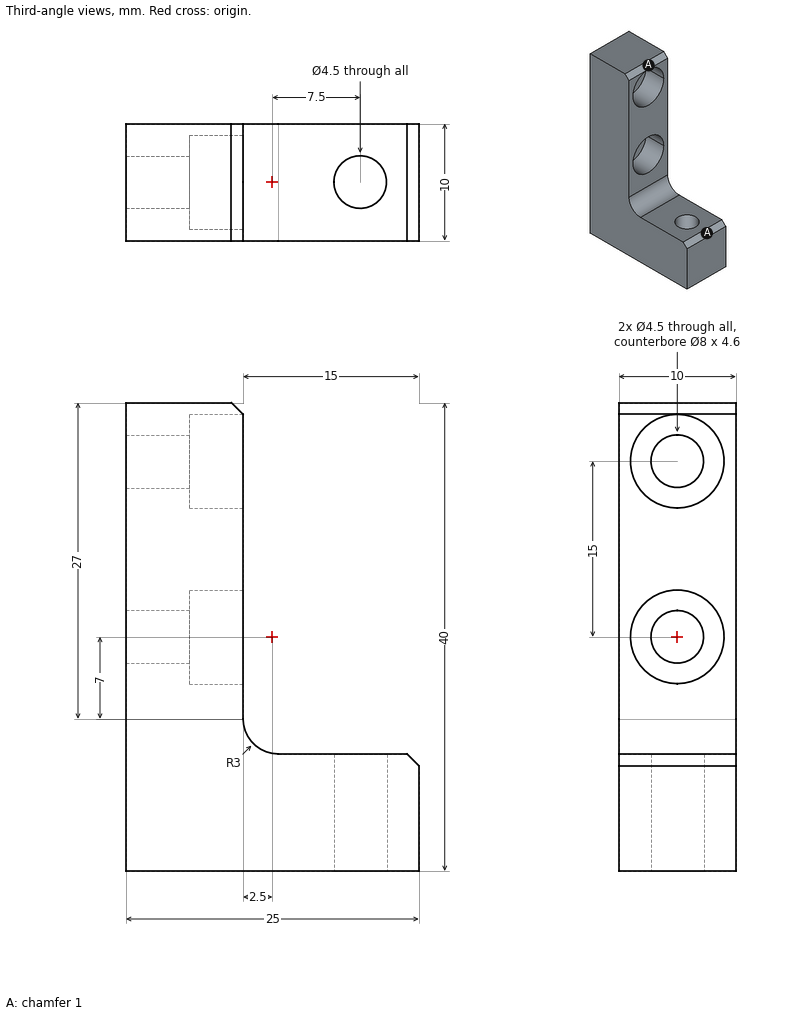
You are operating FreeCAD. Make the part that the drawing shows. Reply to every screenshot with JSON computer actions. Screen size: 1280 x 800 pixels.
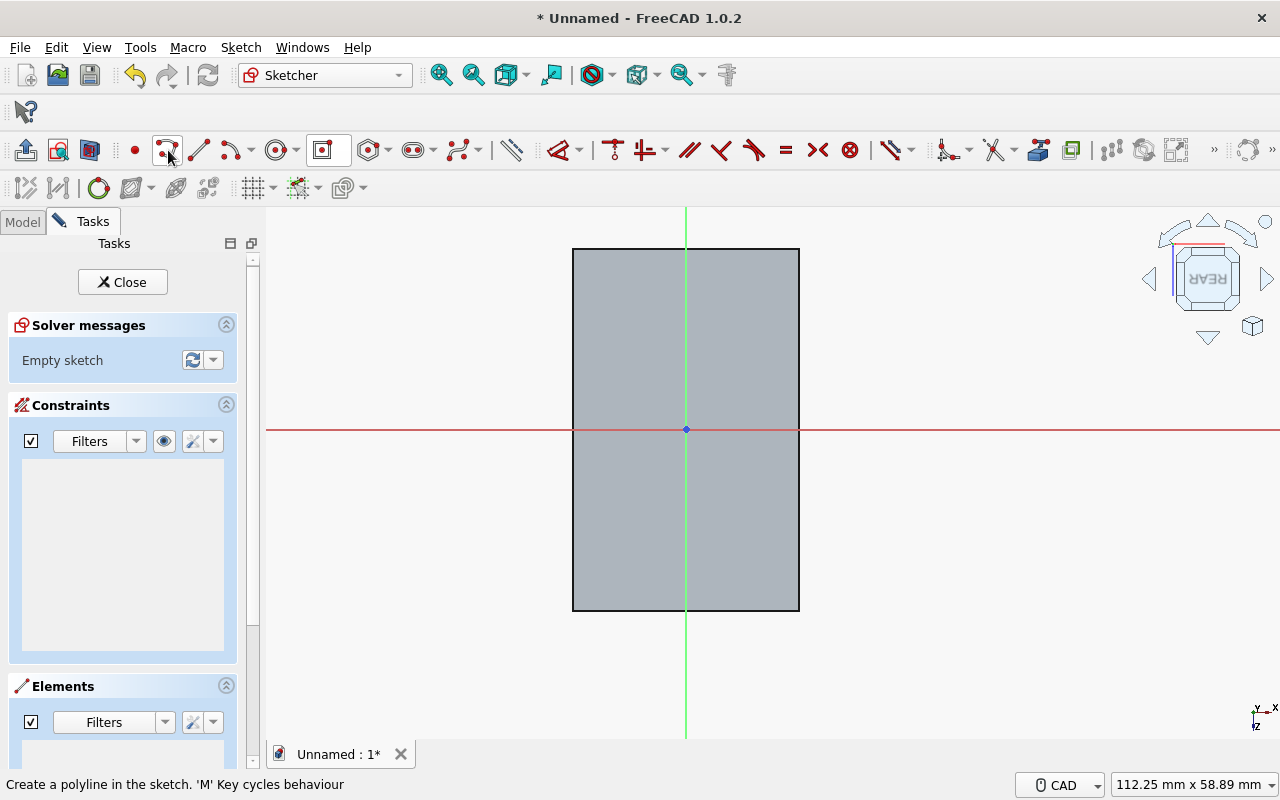
{"action": "left_click", "coordinate": [664, 367]}
{"action": "left_click", "coordinate": [664, 611]}
{"action": "left_click", "coordinate": [799, 611]}
{"action": "left_click", "coordinate": [799, 340]}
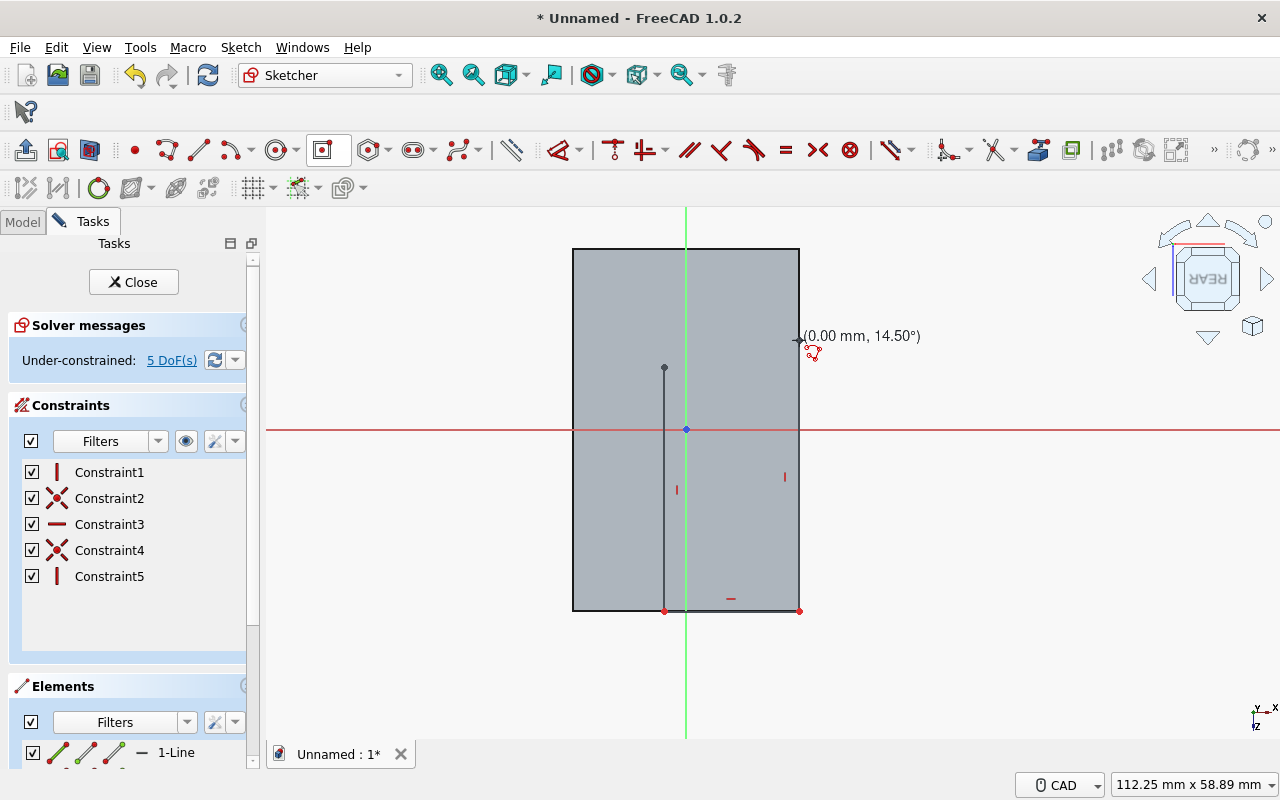
{"action": "scroll", "coordinate": [691, 340], "scroll_direction": "up", "scroll_amount": 7}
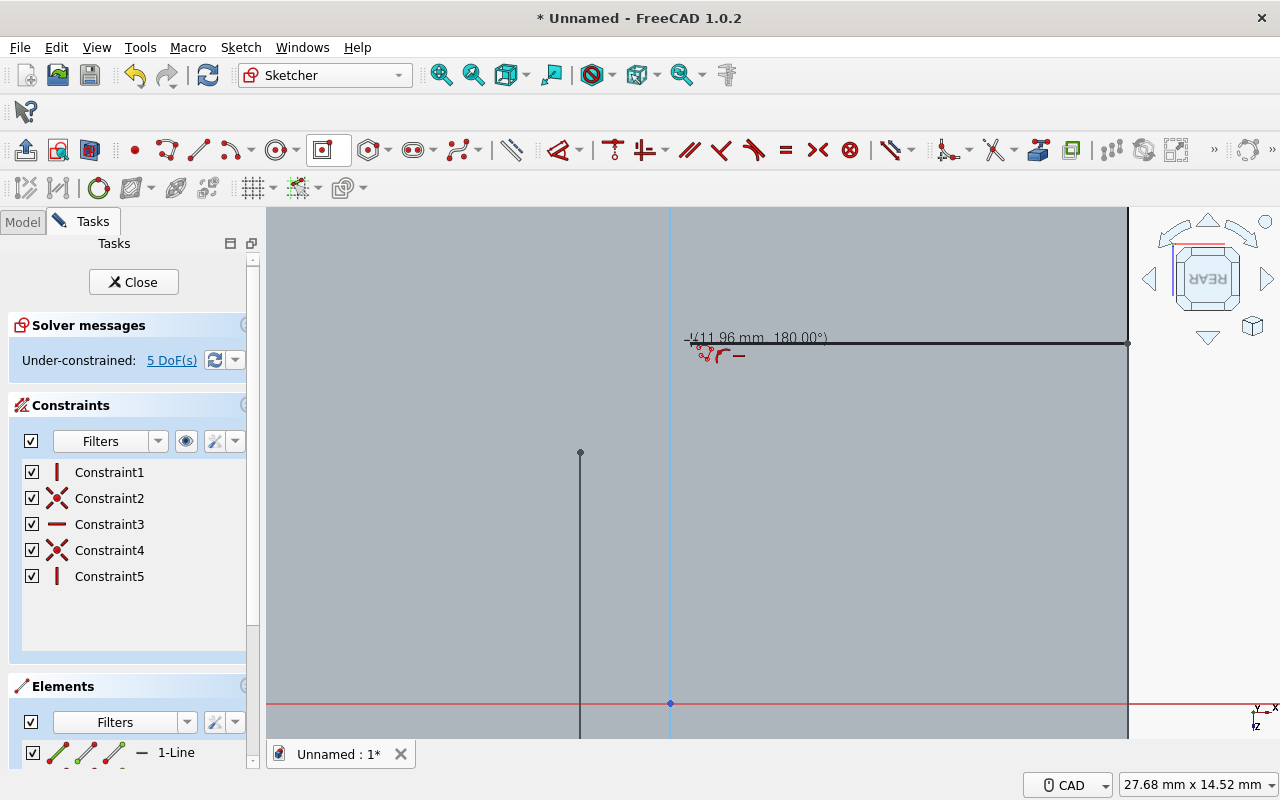
{"action": "left_click", "coordinate": [688, 339]}
{"action": "right_click", "coordinate": [688, 339]}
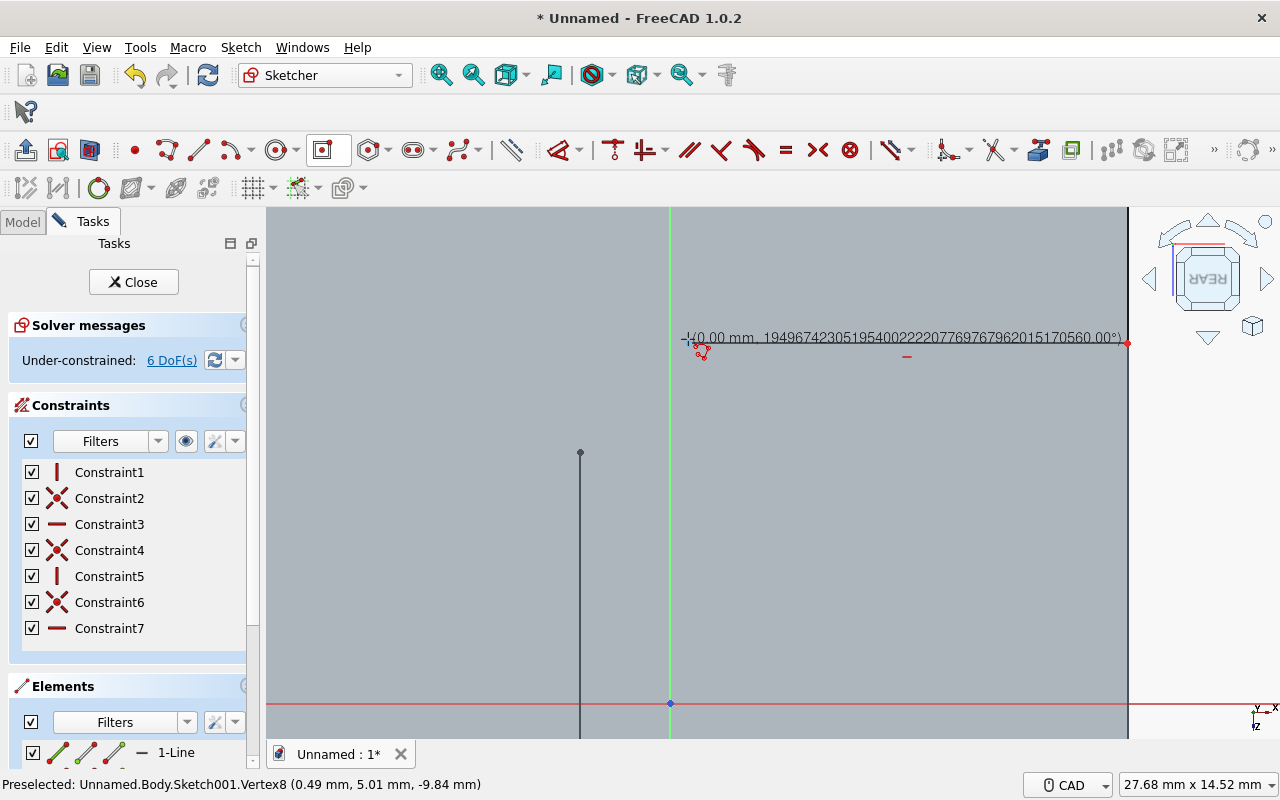
{"action": "left_click", "coordinate": [254, 150]}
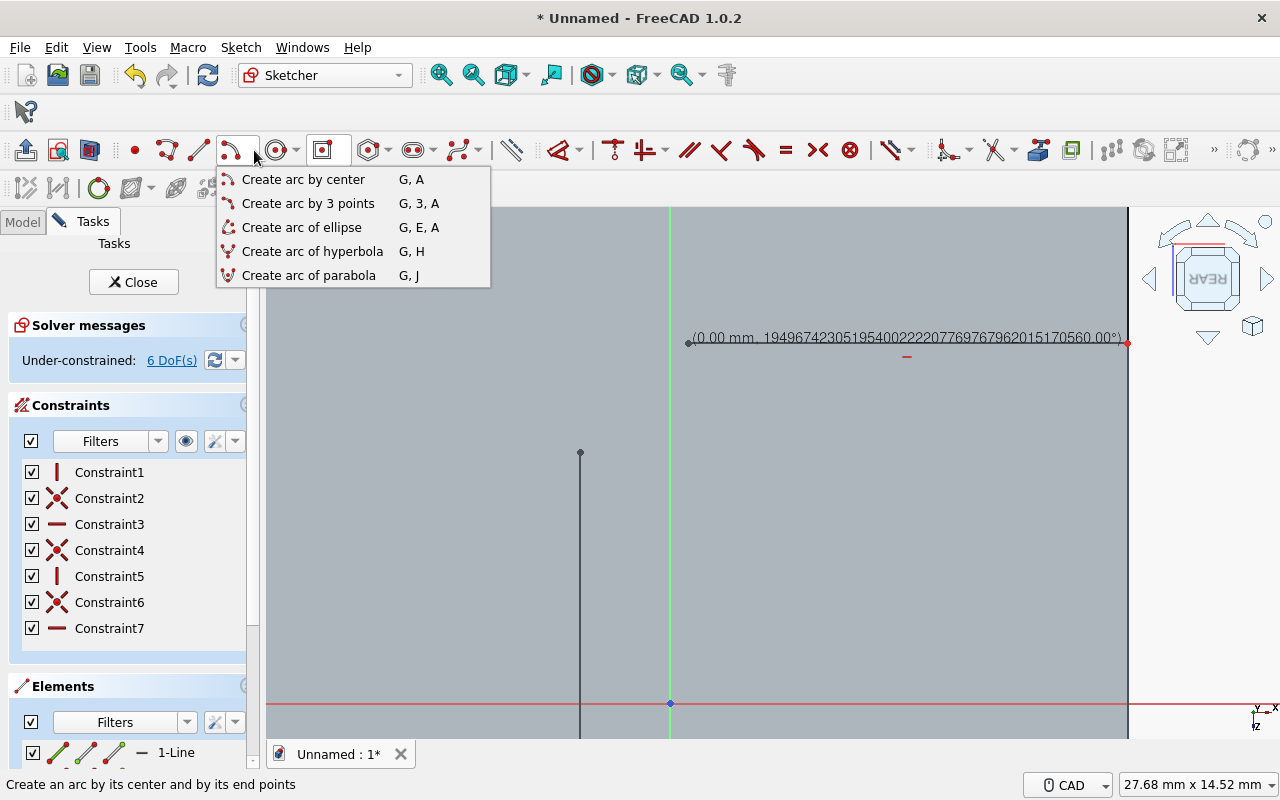
{"action": "left_click", "coordinate": [354, 203]}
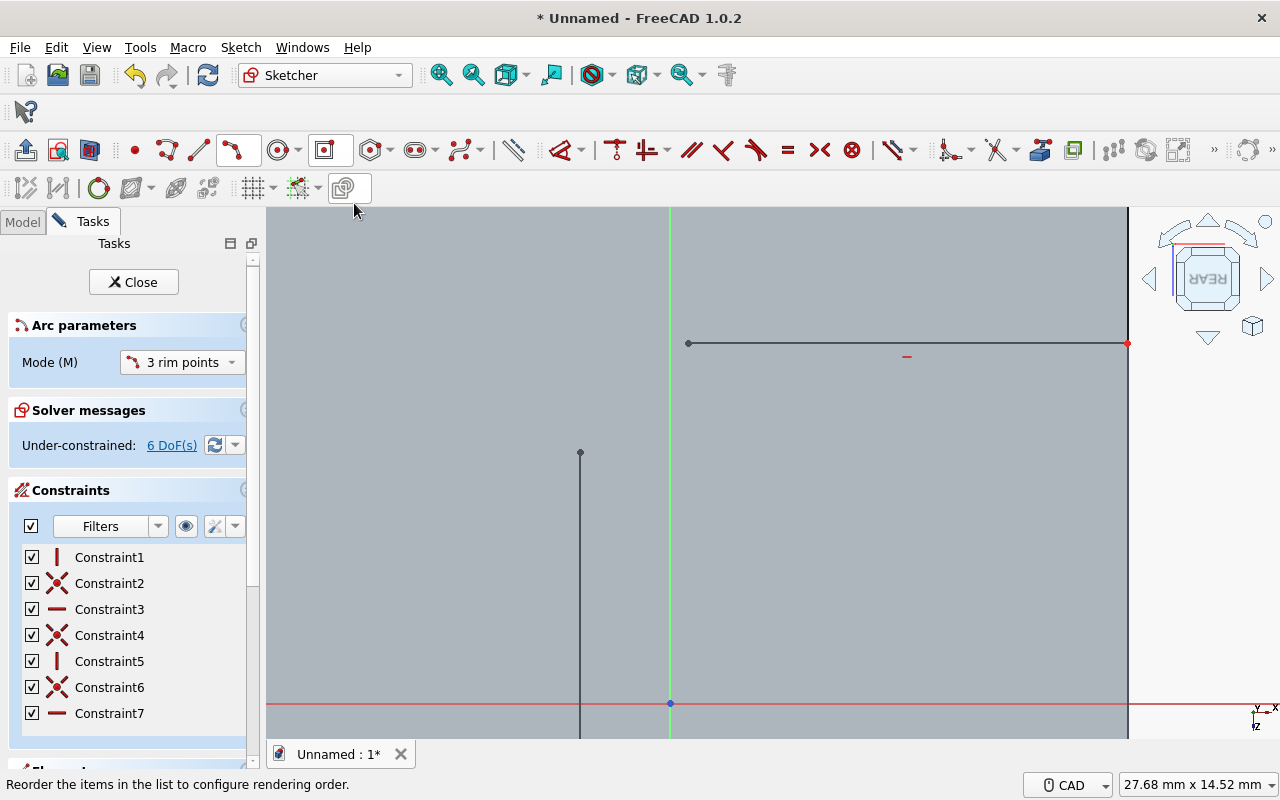
{"action": "left_click", "coordinate": [688, 343]}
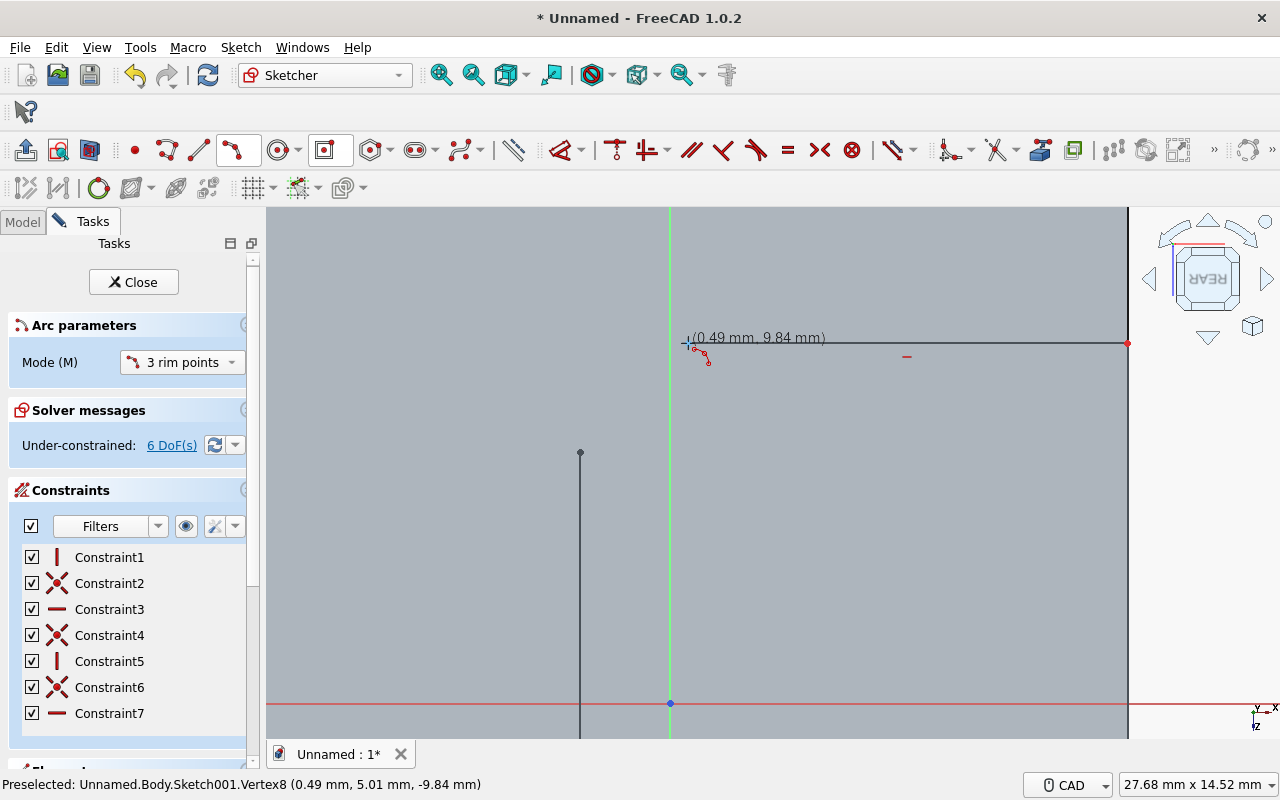
{"action": "scroll", "coordinate": [640, 295], "scroll_direction": "down", "scroll_amount": 6}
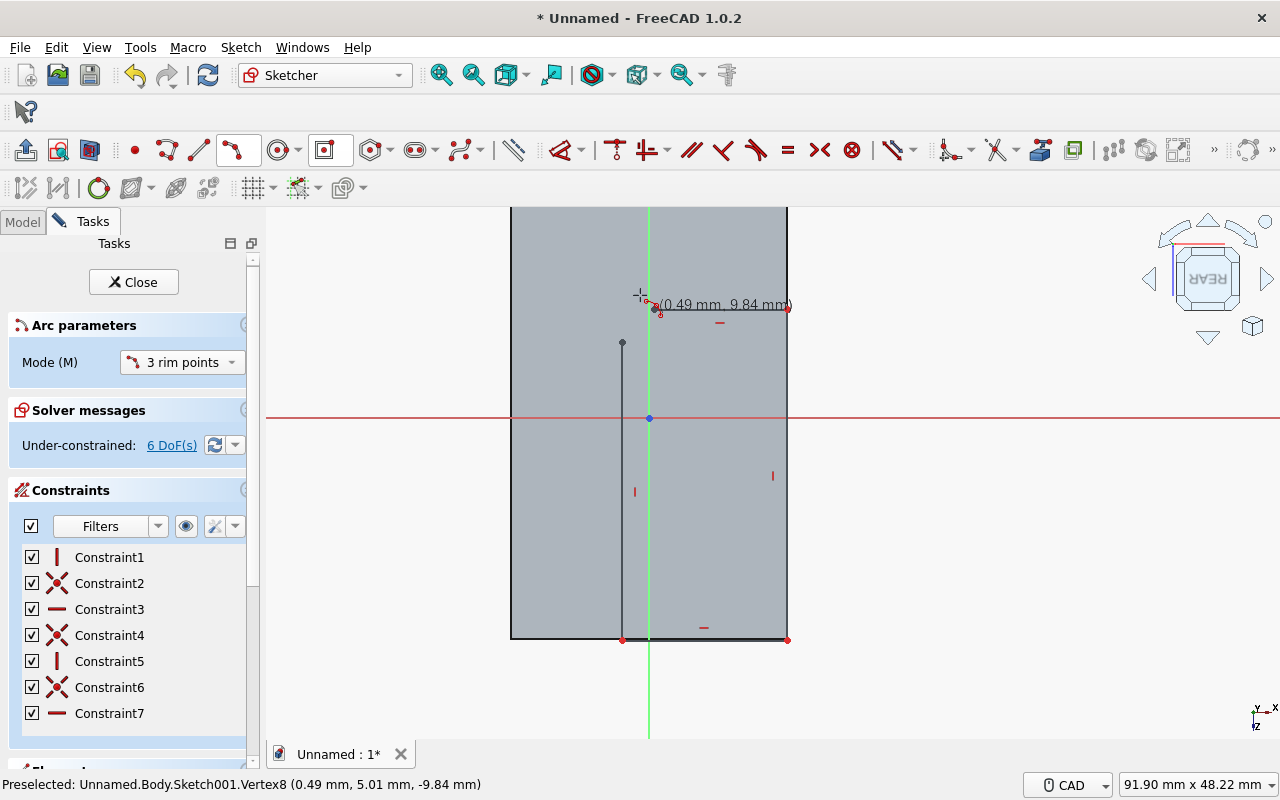
{"action": "left_click", "coordinate": [622, 343]}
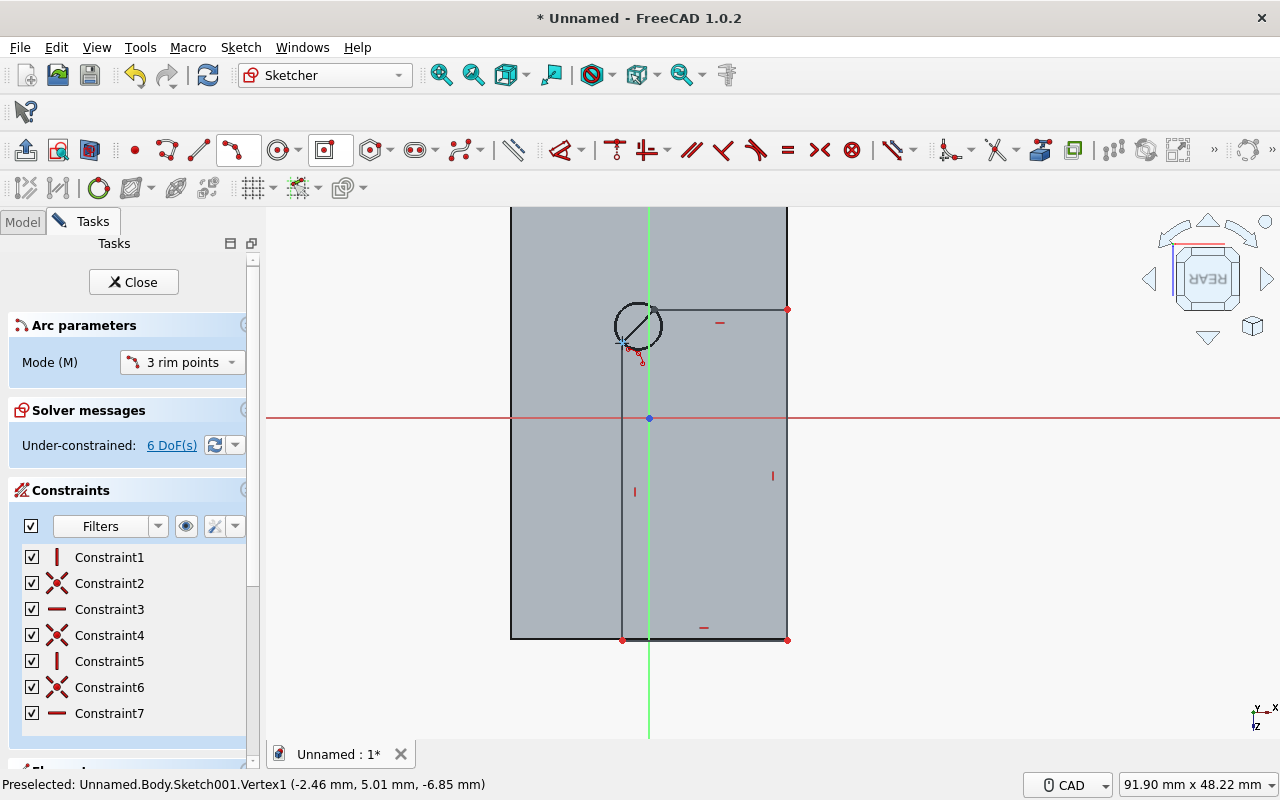
{"action": "scroll", "coordinate": [631, 318], "scroll_direction": "up", "scroll_amount": 3}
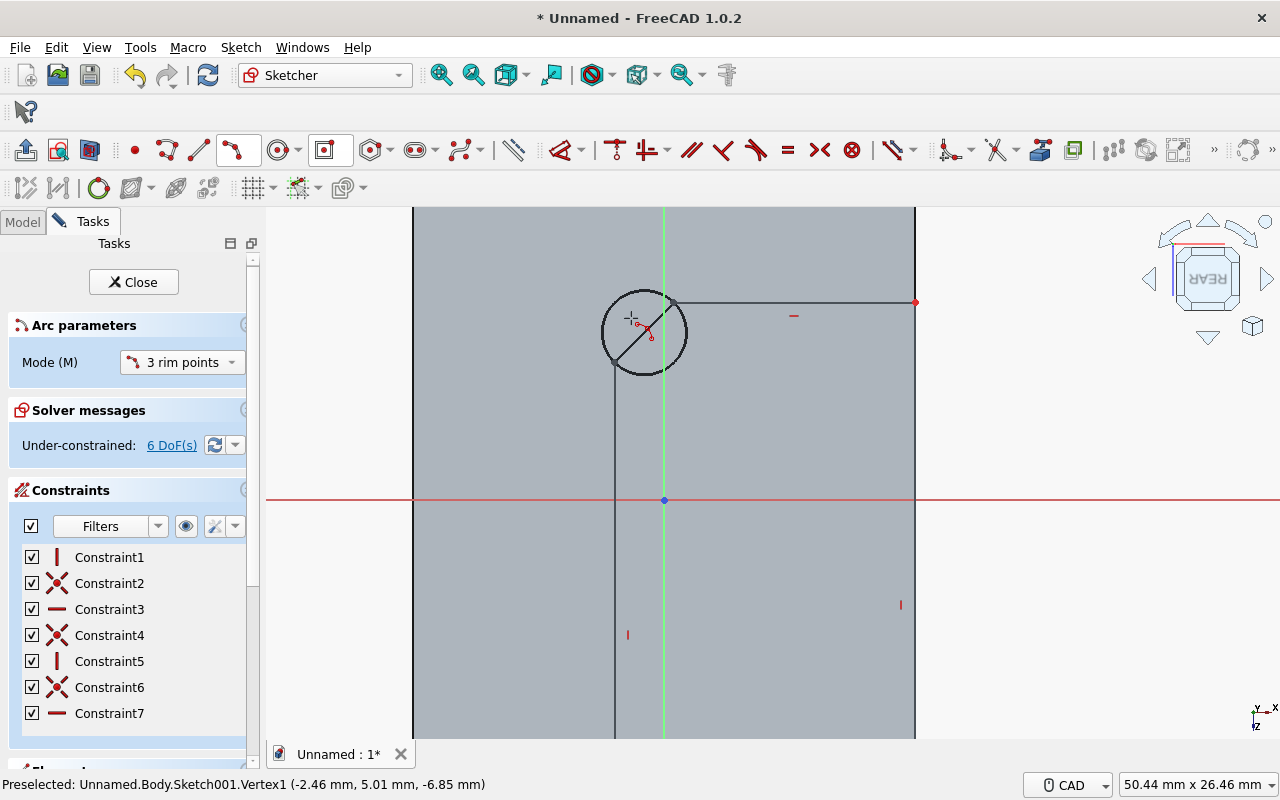
{"action": "left_click", "coordinate": [632, 317]}
{"action": "key", "text": "Escape"}